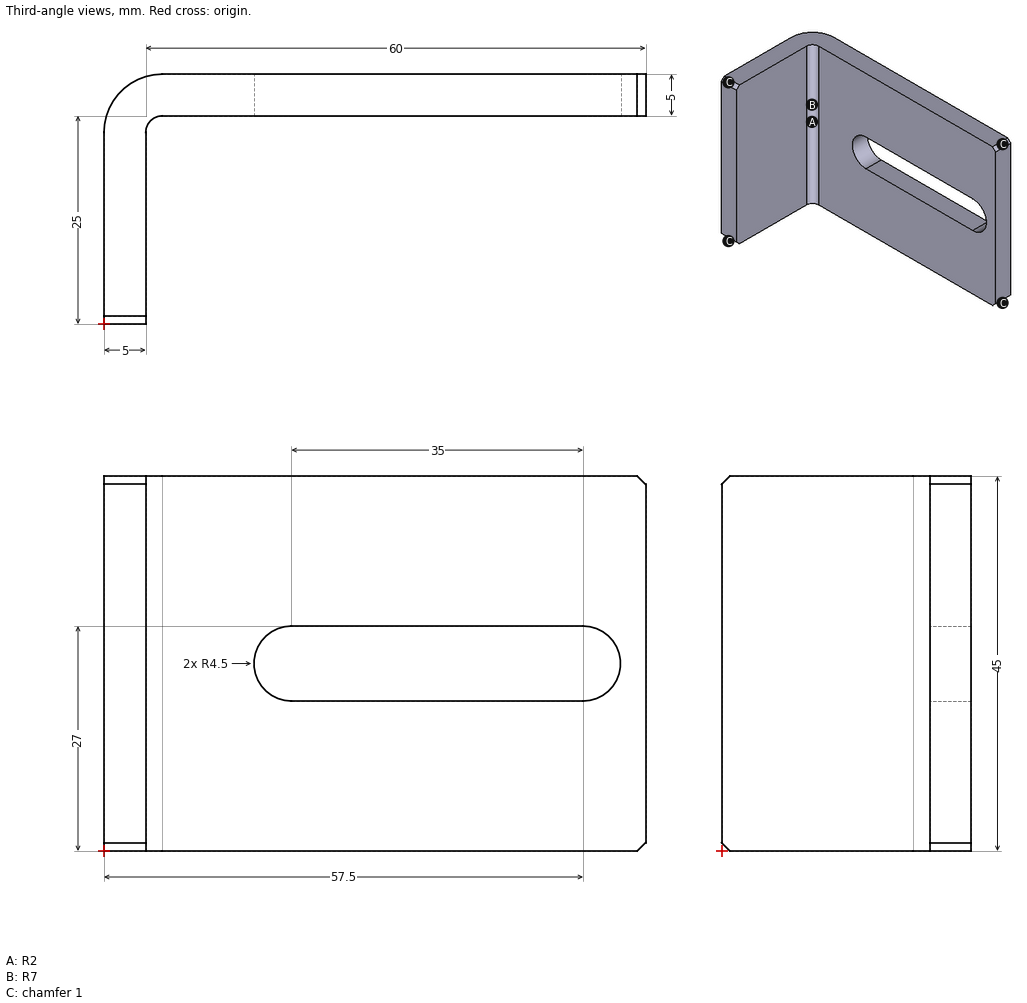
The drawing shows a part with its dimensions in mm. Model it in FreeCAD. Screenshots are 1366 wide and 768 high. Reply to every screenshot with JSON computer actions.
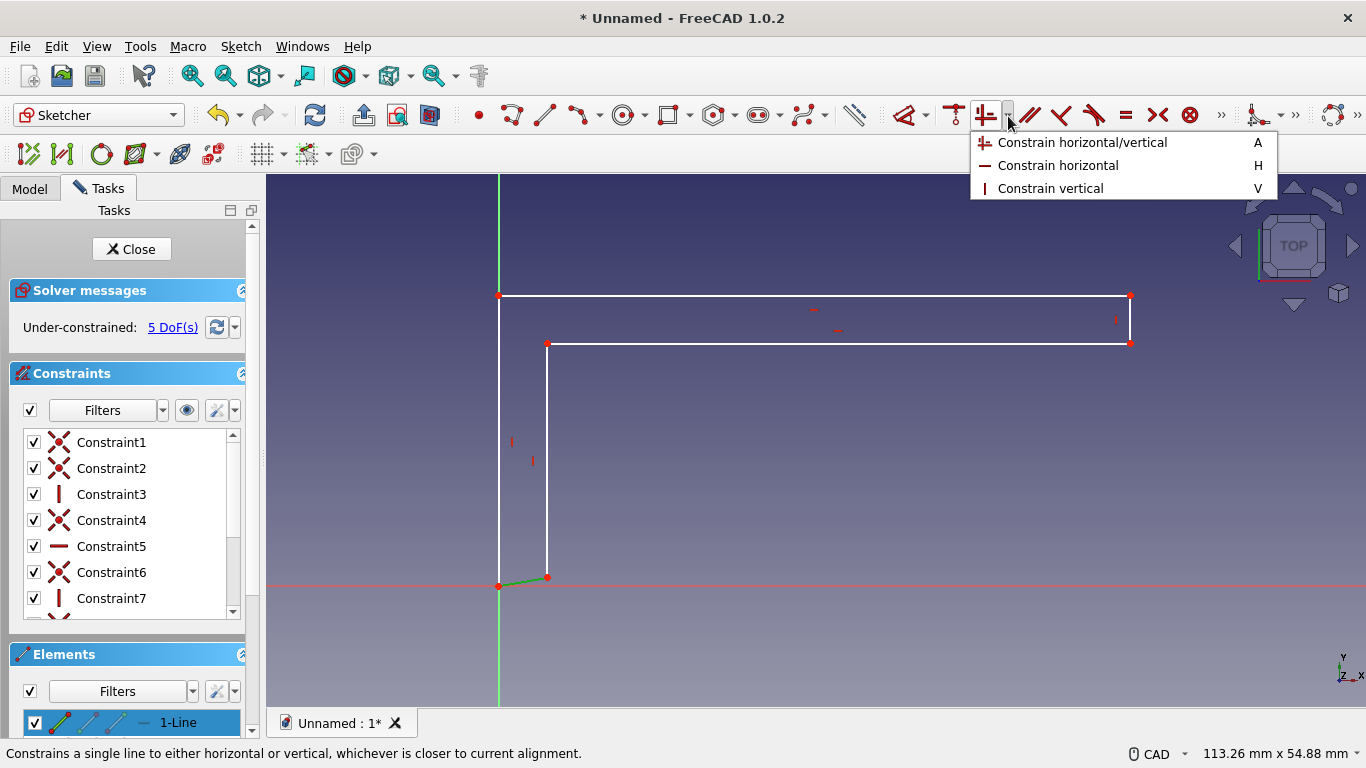
{"action": "left_click", "coordinate": [1124, 166]}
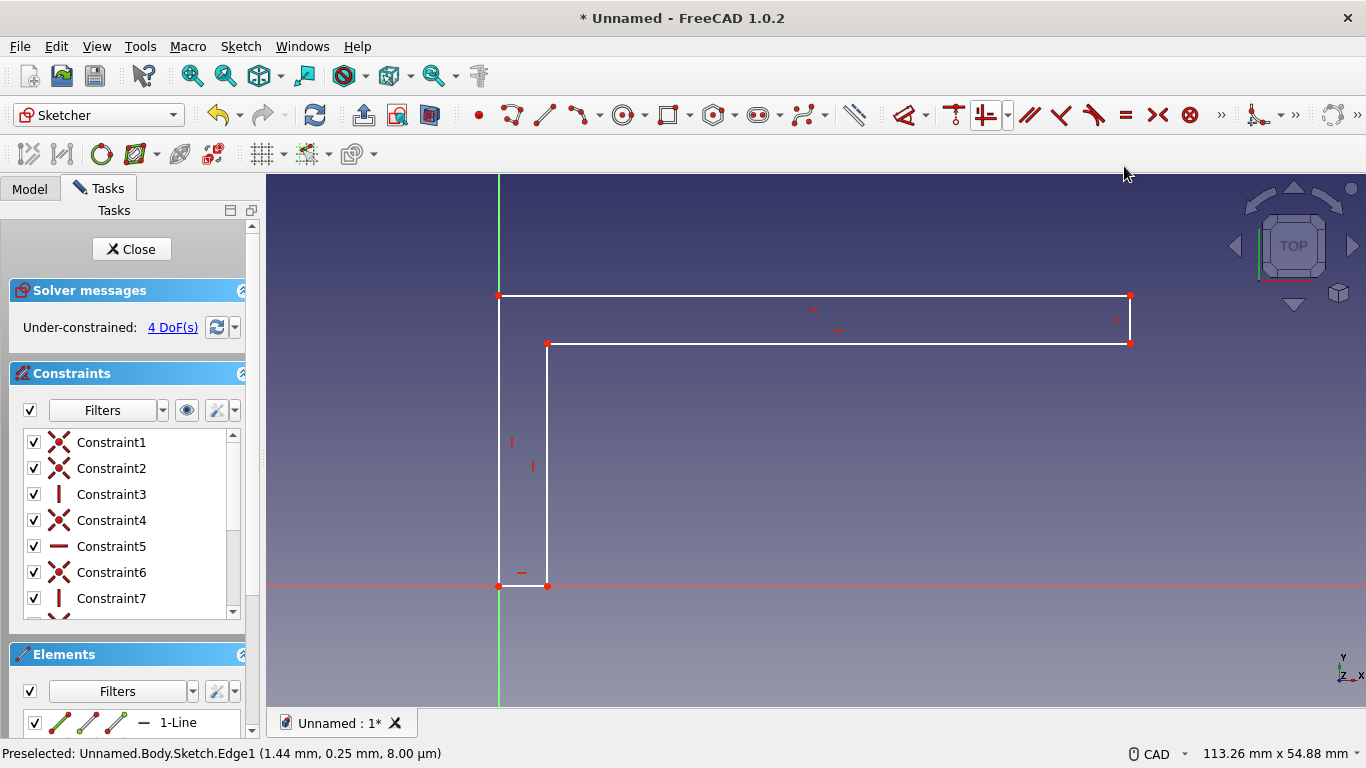
{"action": "left_click", "coordinate": [904, 116]}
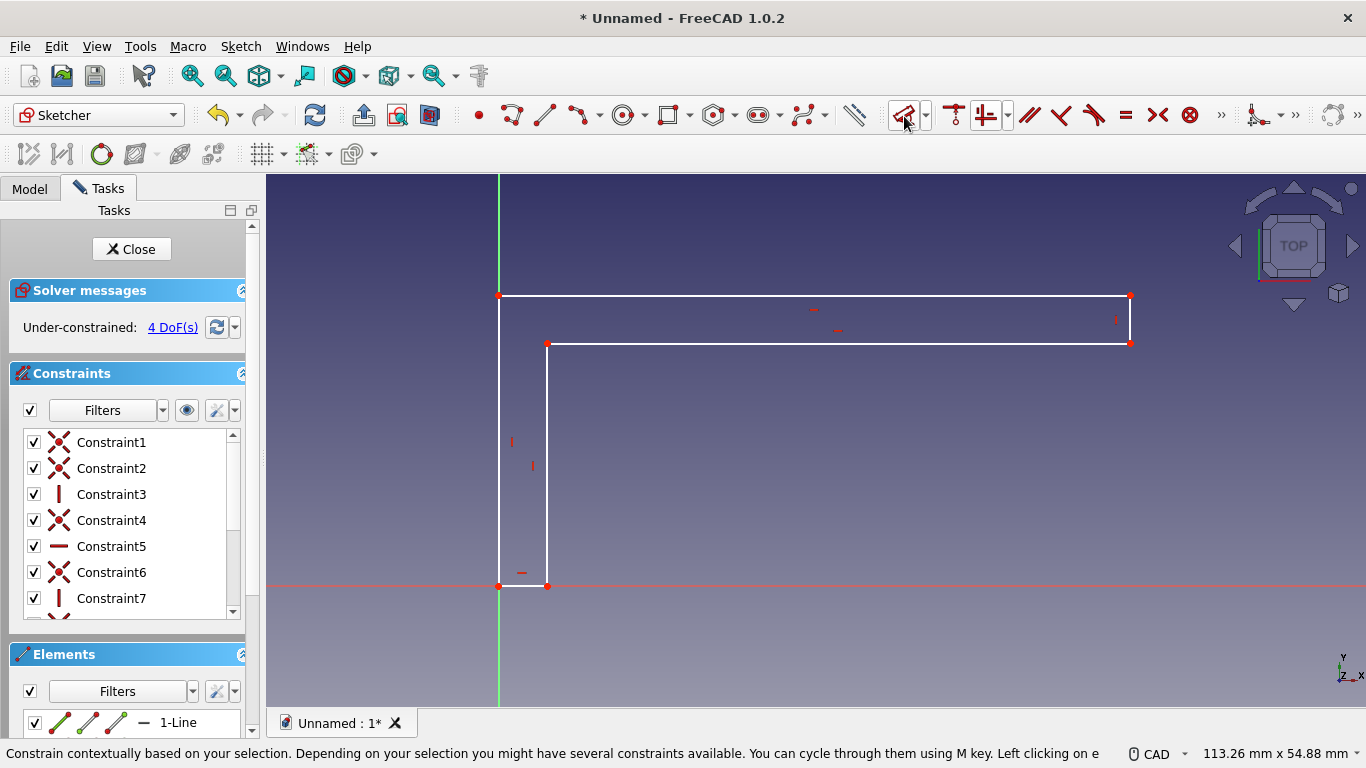
{"action": "left_click", "coordinate": [513, 586]}
{"action": "left_click", "coordinate": [523, 620]}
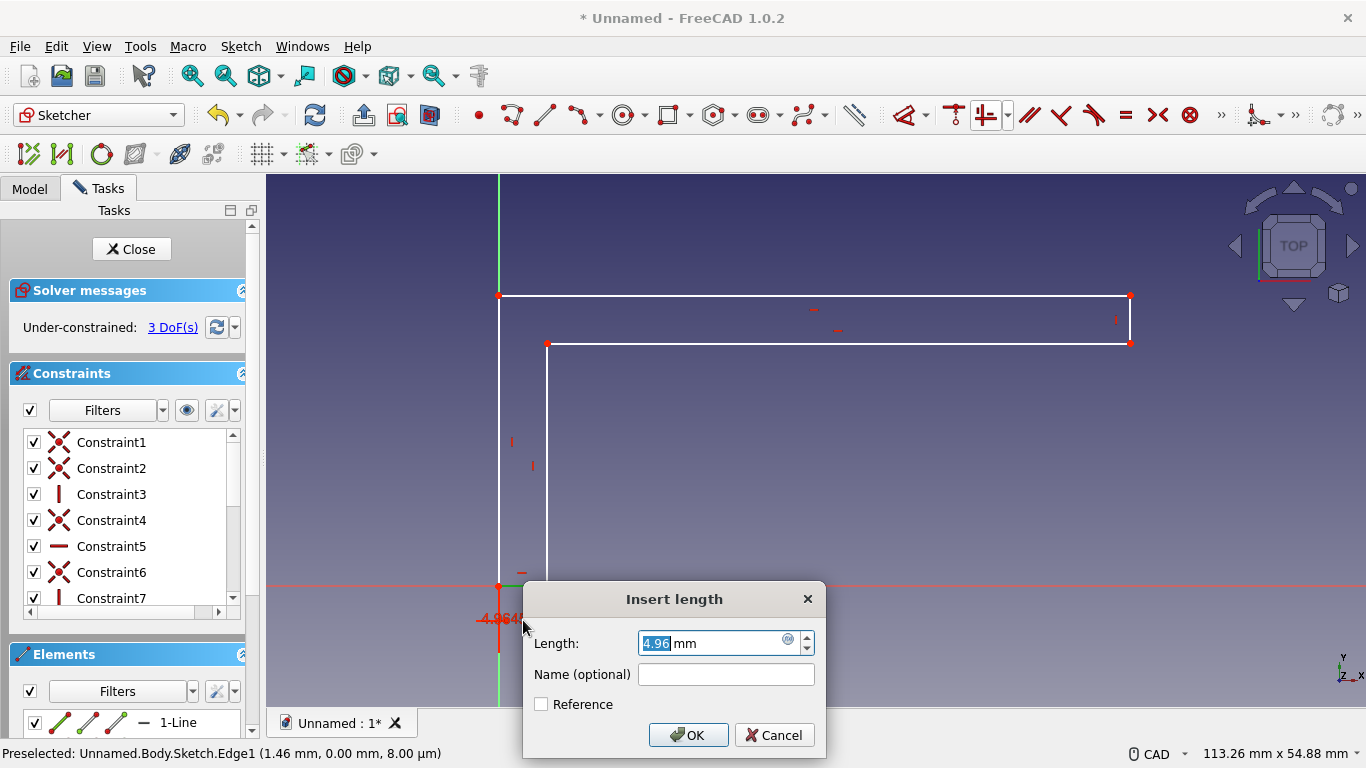
{"action": "type", "text": "5"}
{"action": "key", "text": "Return"}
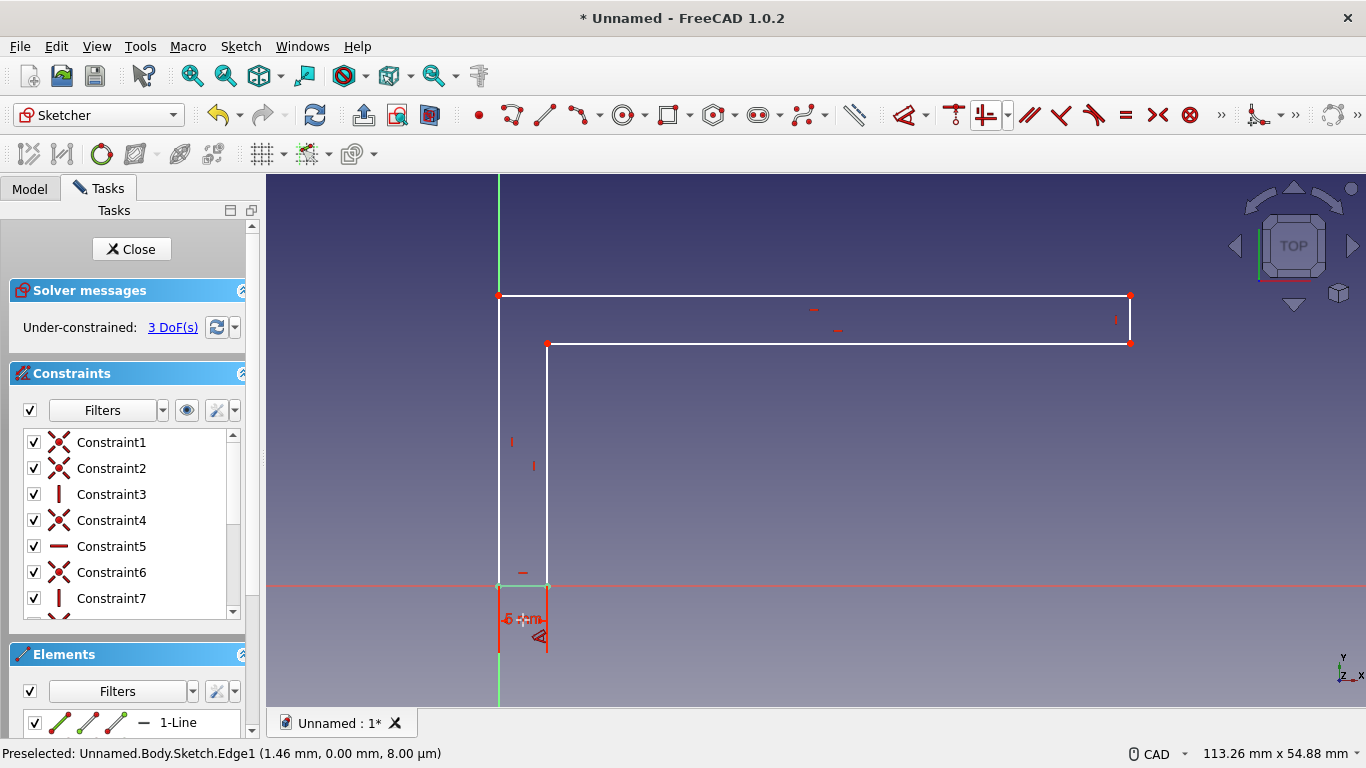
{"action": "left_click", "coordinate": [1130, 330]}
{"action": "left_click", "coordinate": [1164, 320]}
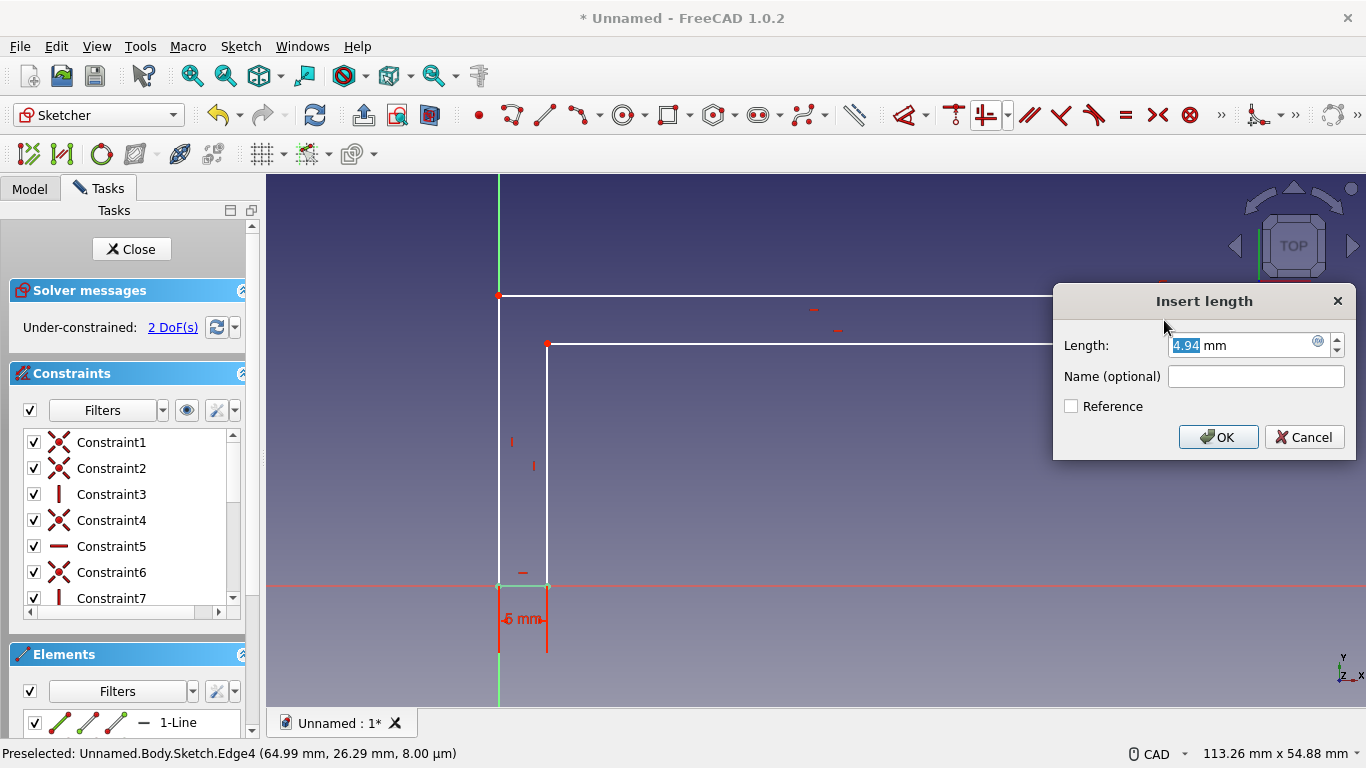
{"action": "type", "text": "5"}
{"action": "key", "text": "Return"}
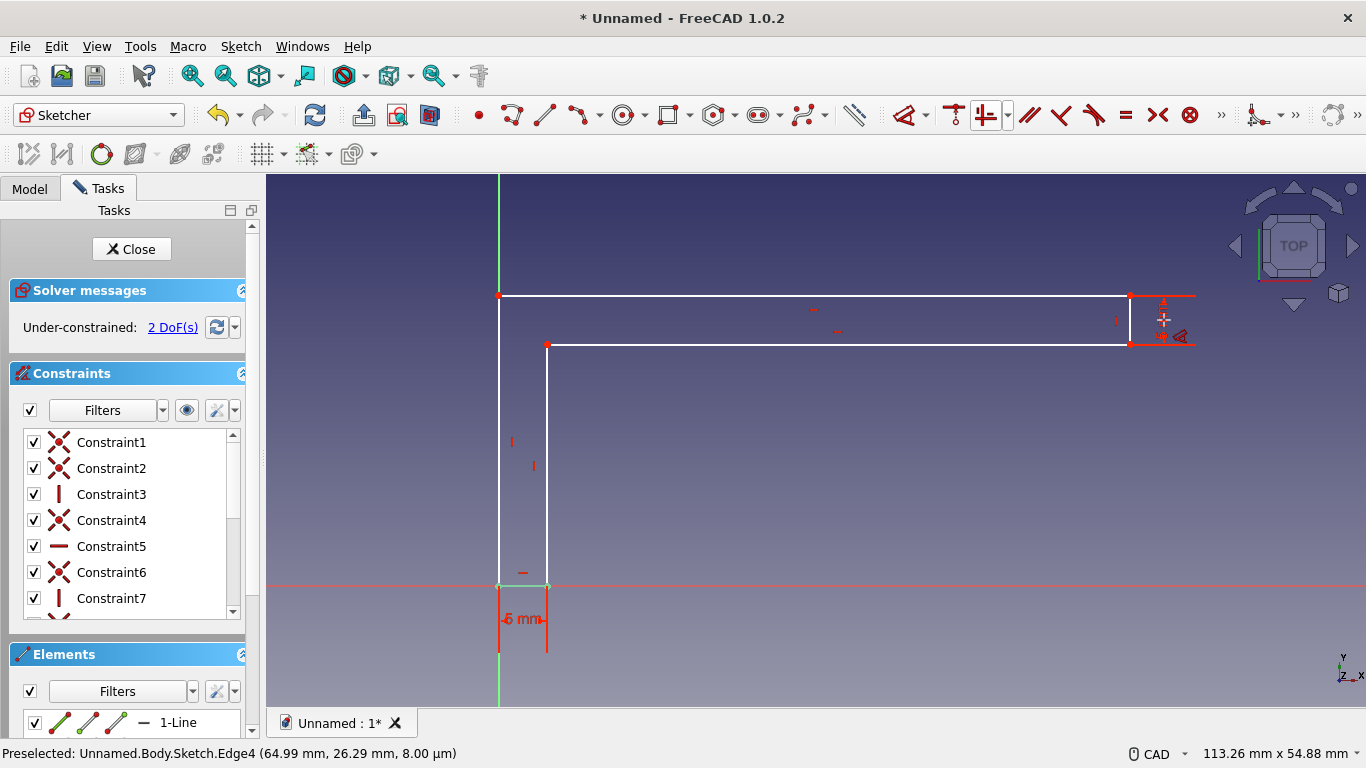
{"action": "left_click", "coordinate": [547, 514]}
{"action": "left_click", "coordinate": [513, 465]}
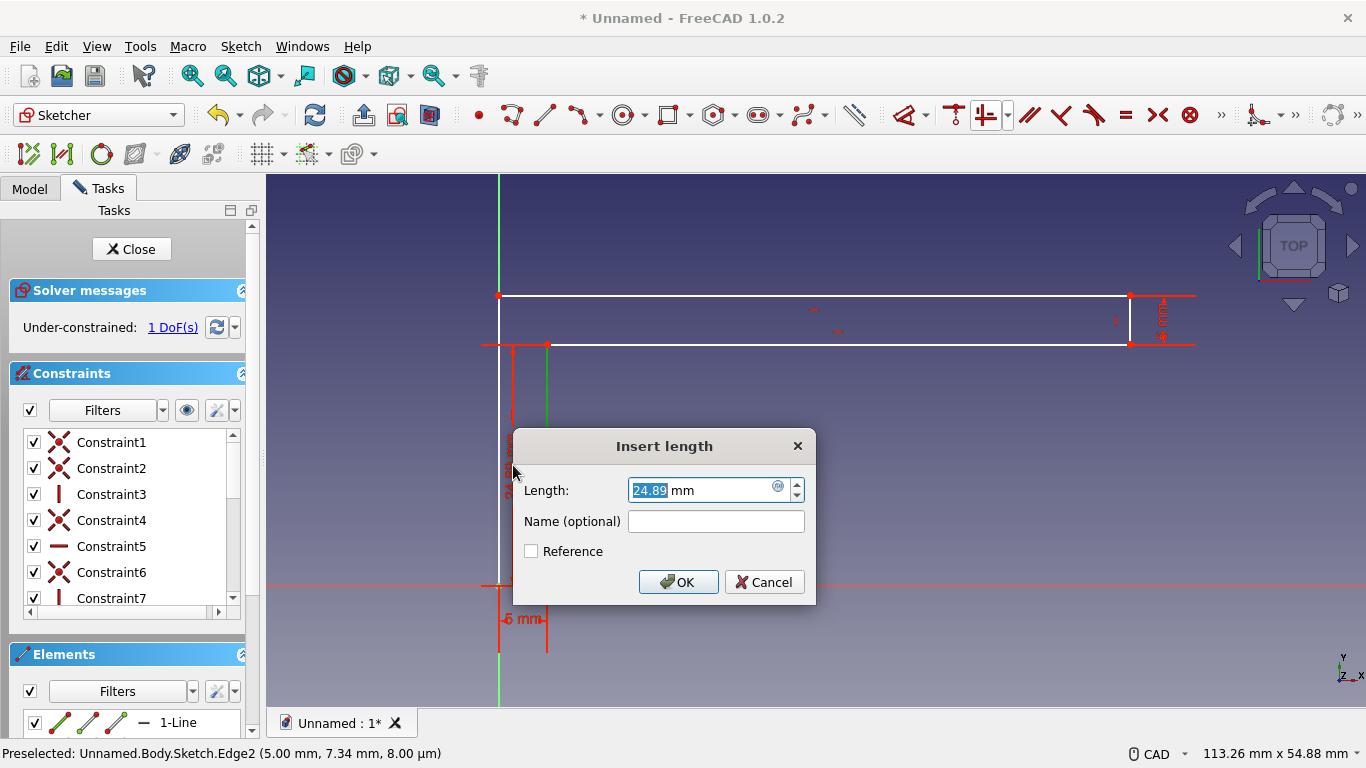
{"action": "type", "text": "25"}
{"action": "key", "text": "Return"}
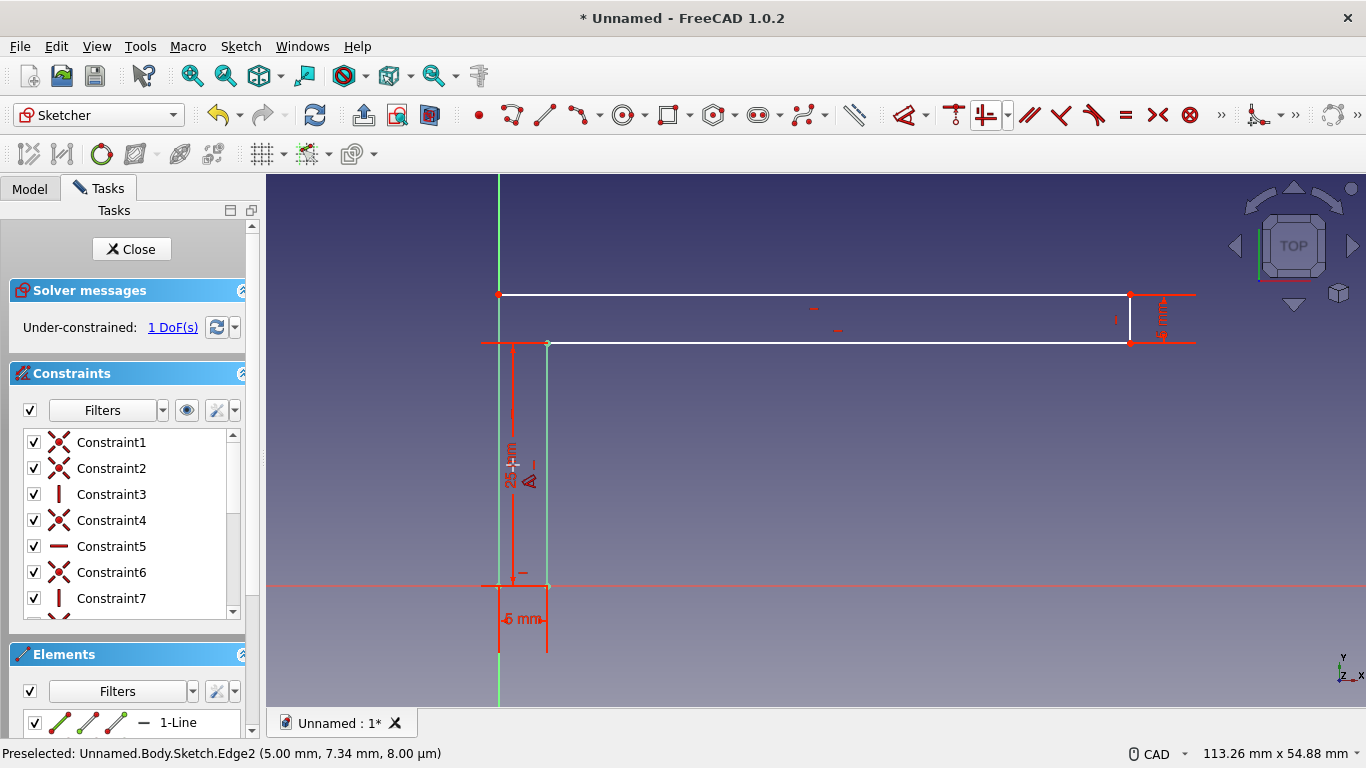
{"action": "left_click", "coordinate": [722, 343]}
{"action": "left_click", "coordinate": [839, 309]}